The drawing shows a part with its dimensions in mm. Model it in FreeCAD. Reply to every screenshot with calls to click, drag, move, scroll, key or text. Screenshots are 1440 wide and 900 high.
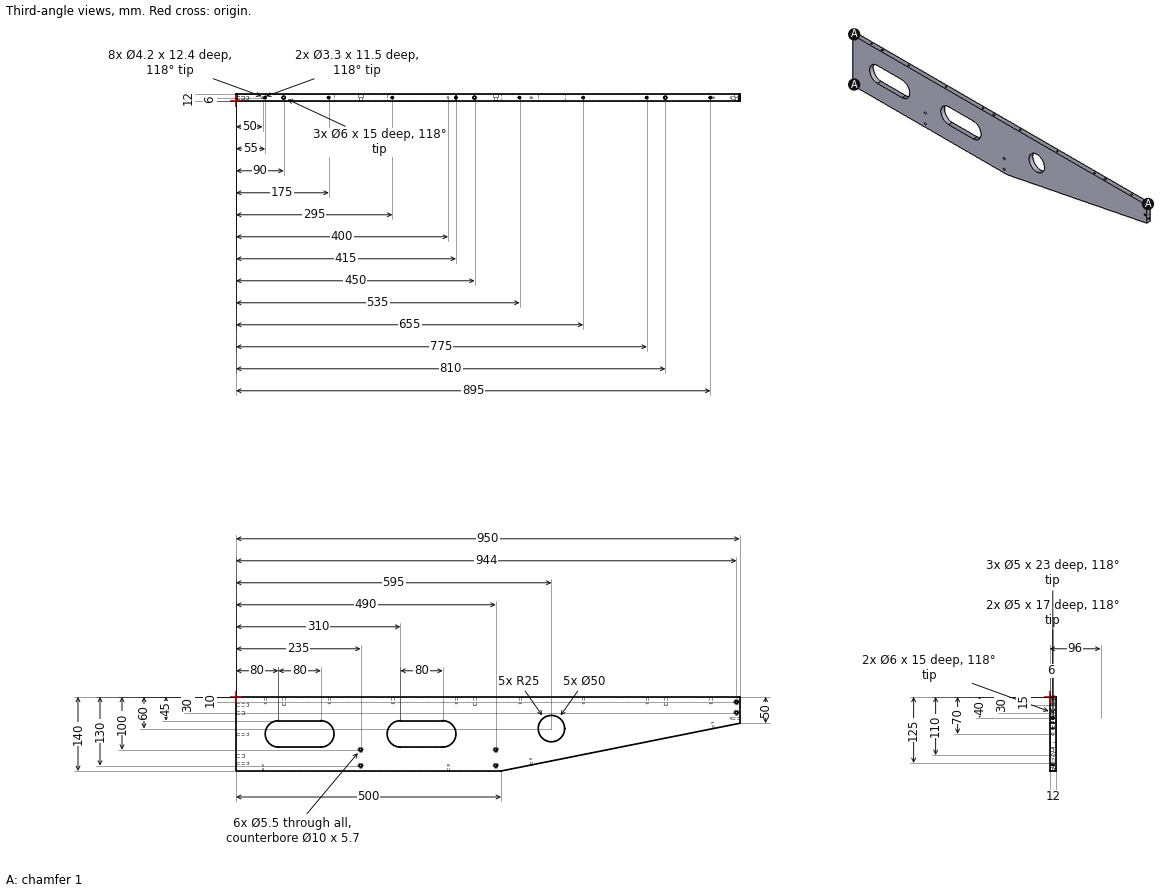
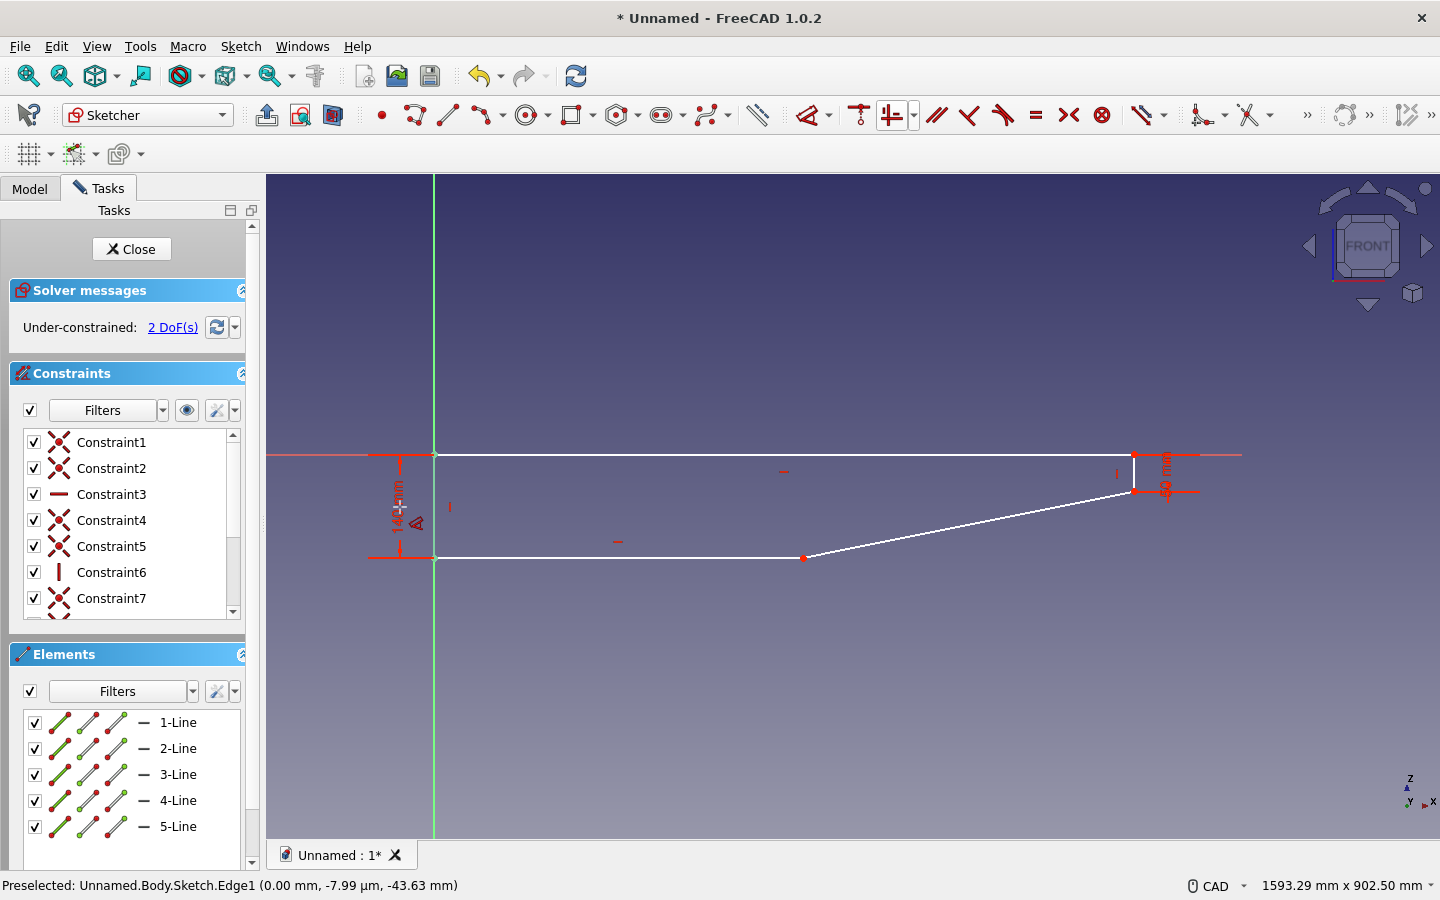
click(545, 558)
click(619, 592)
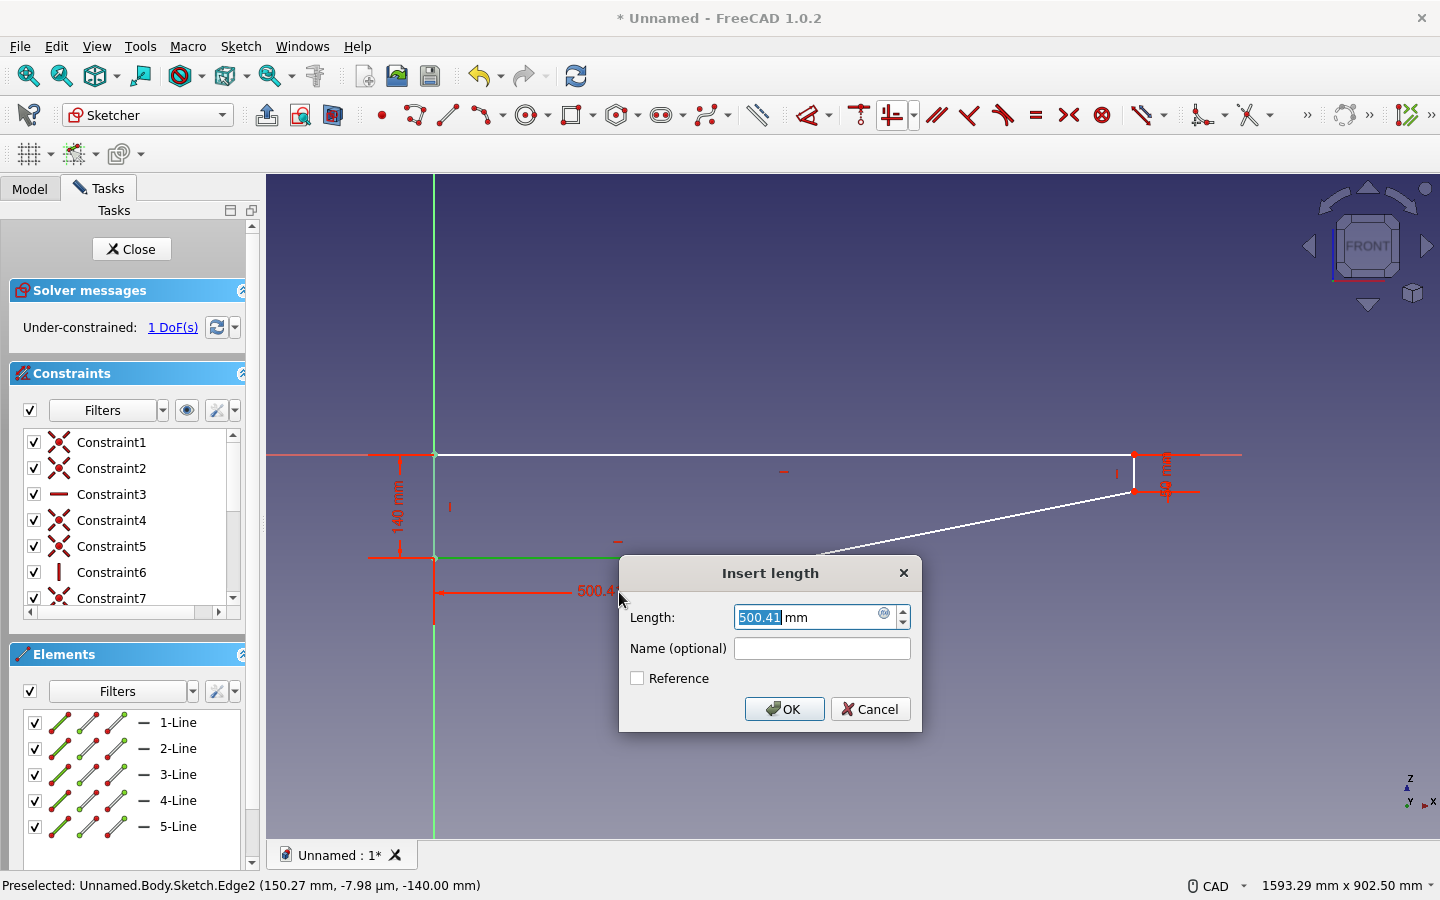
text(500)
key(Return)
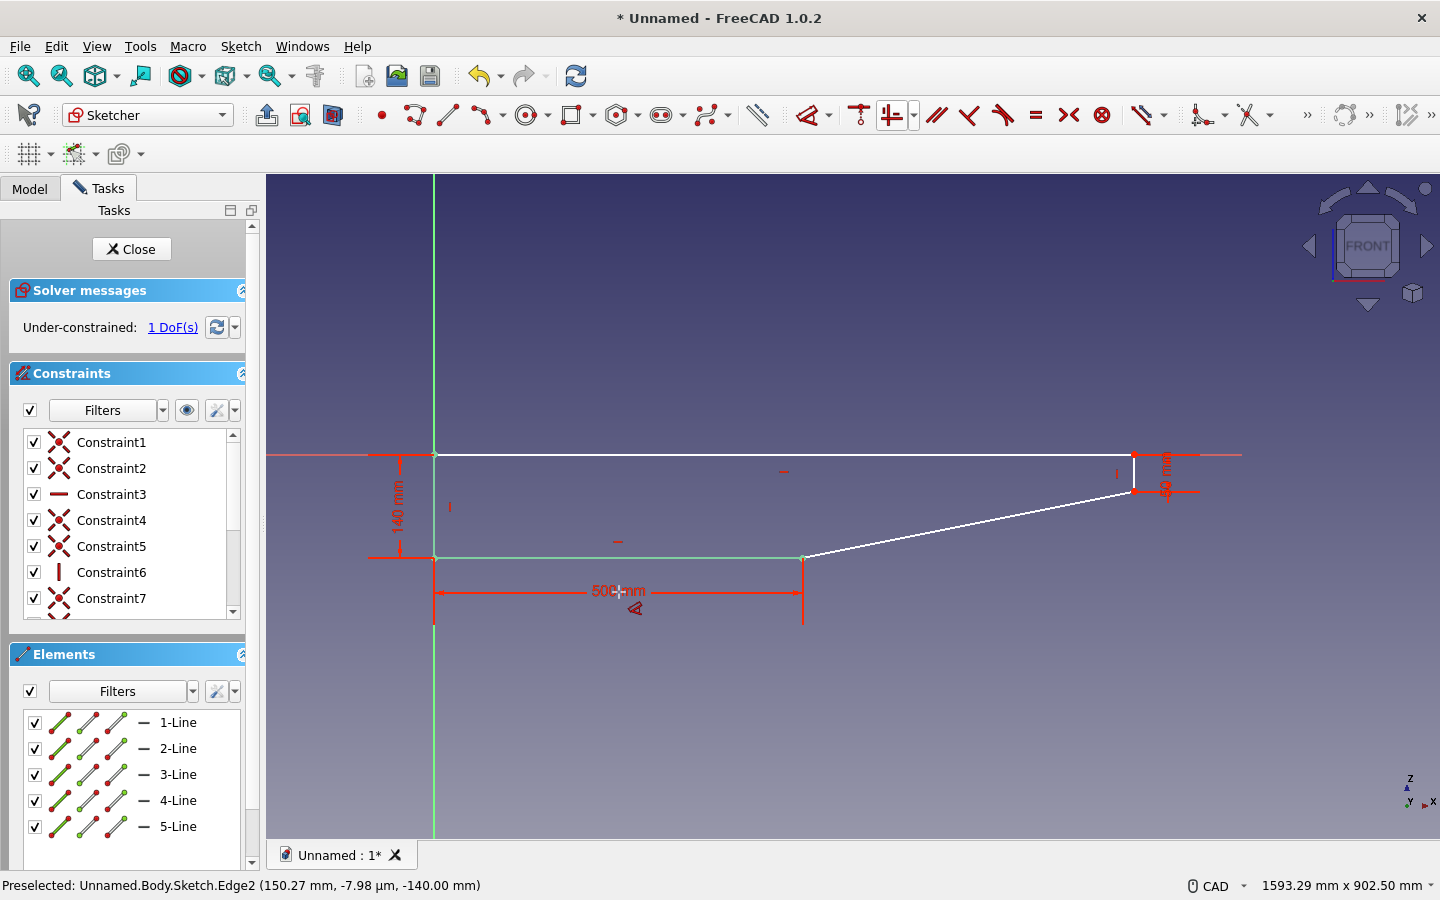
click(924, 455)
click(784, 421)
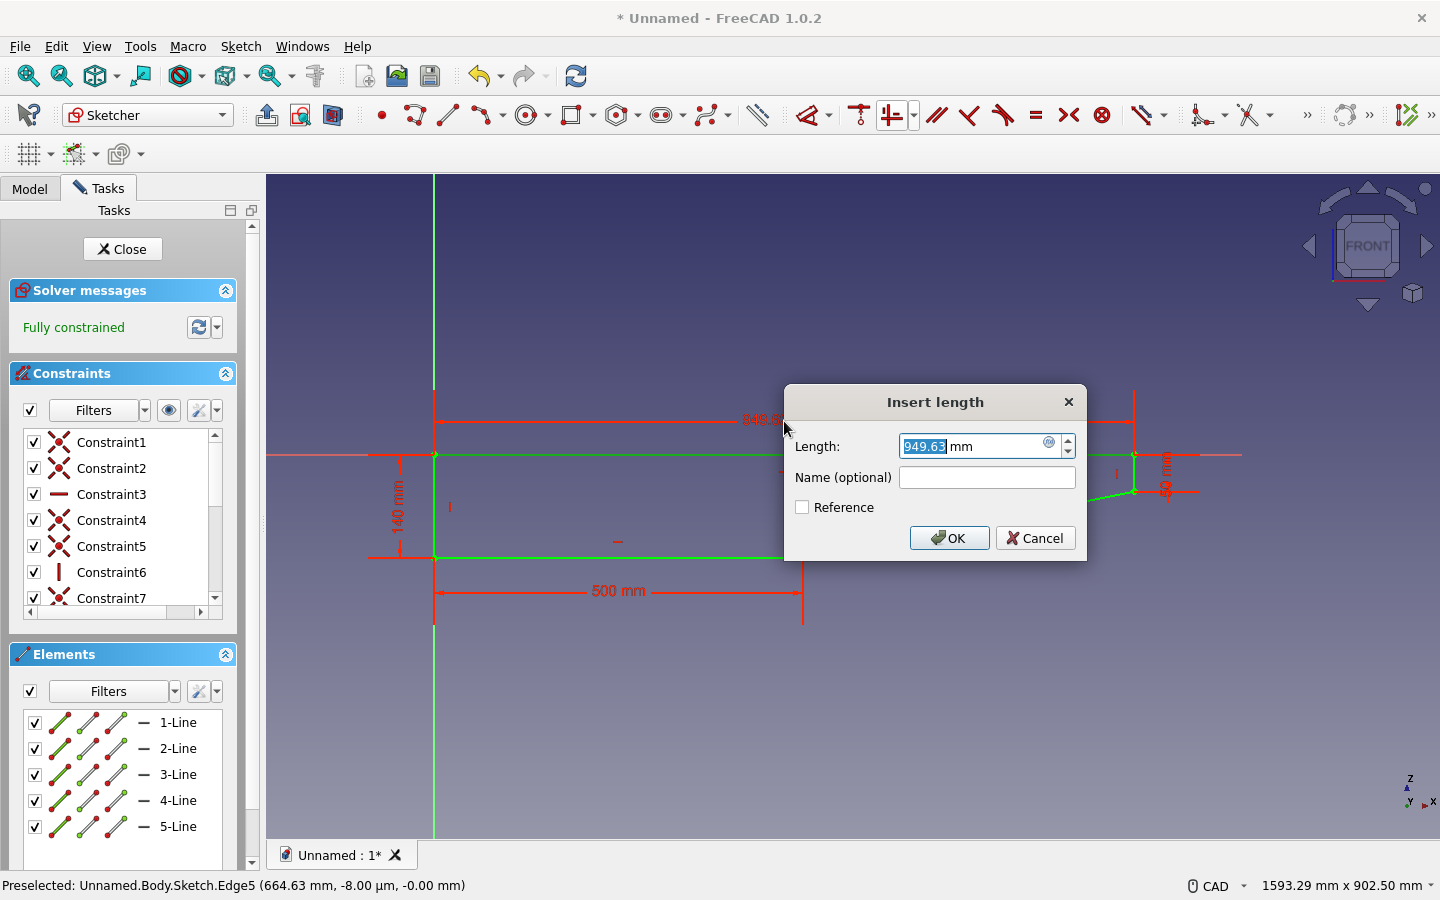
text(950)
key(Return)
key(Escape)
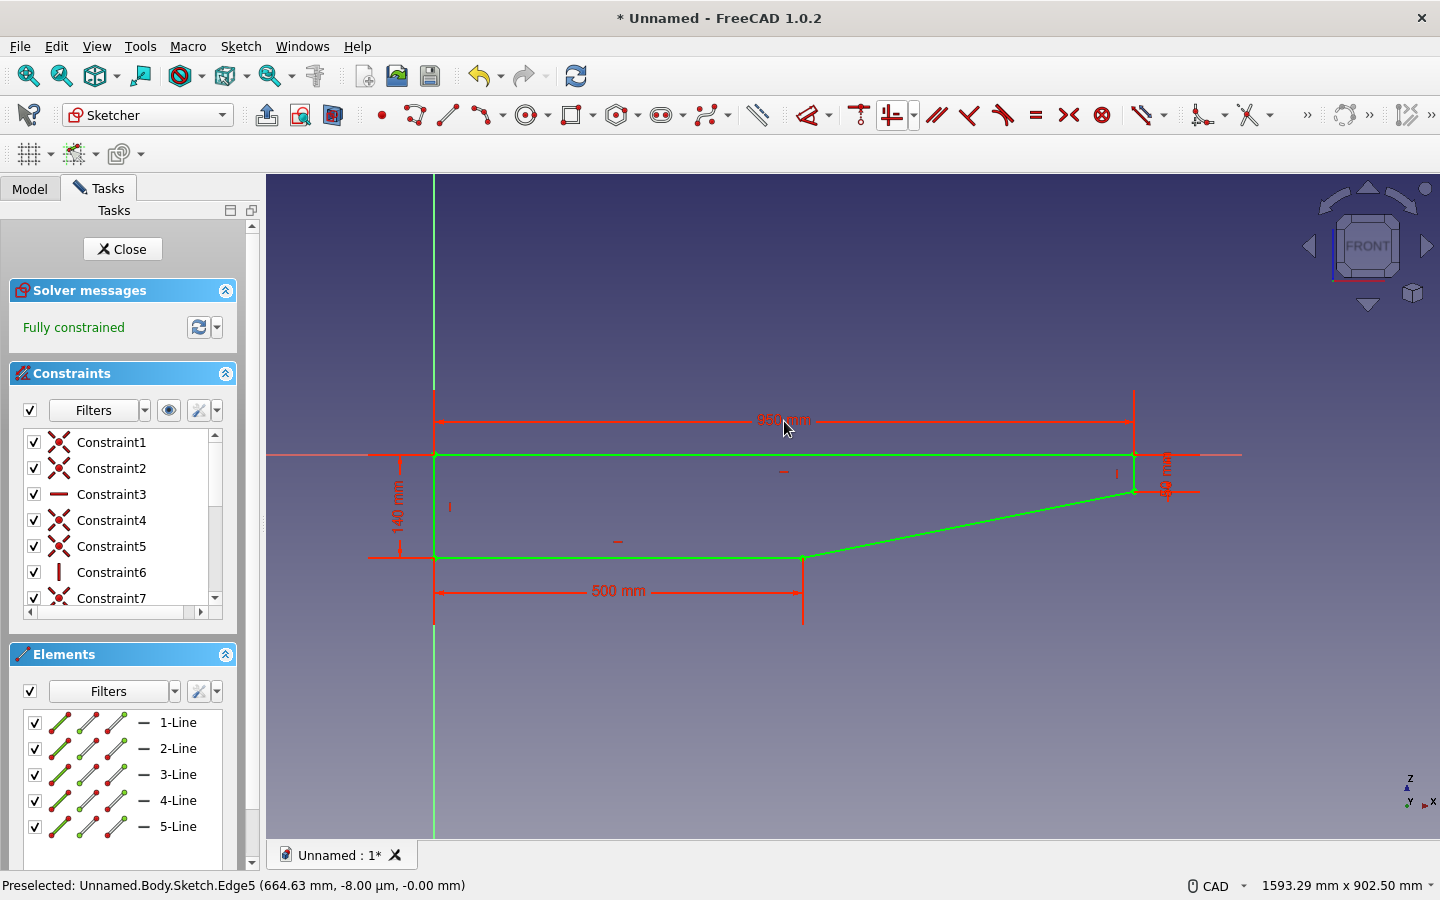
click(123, 249)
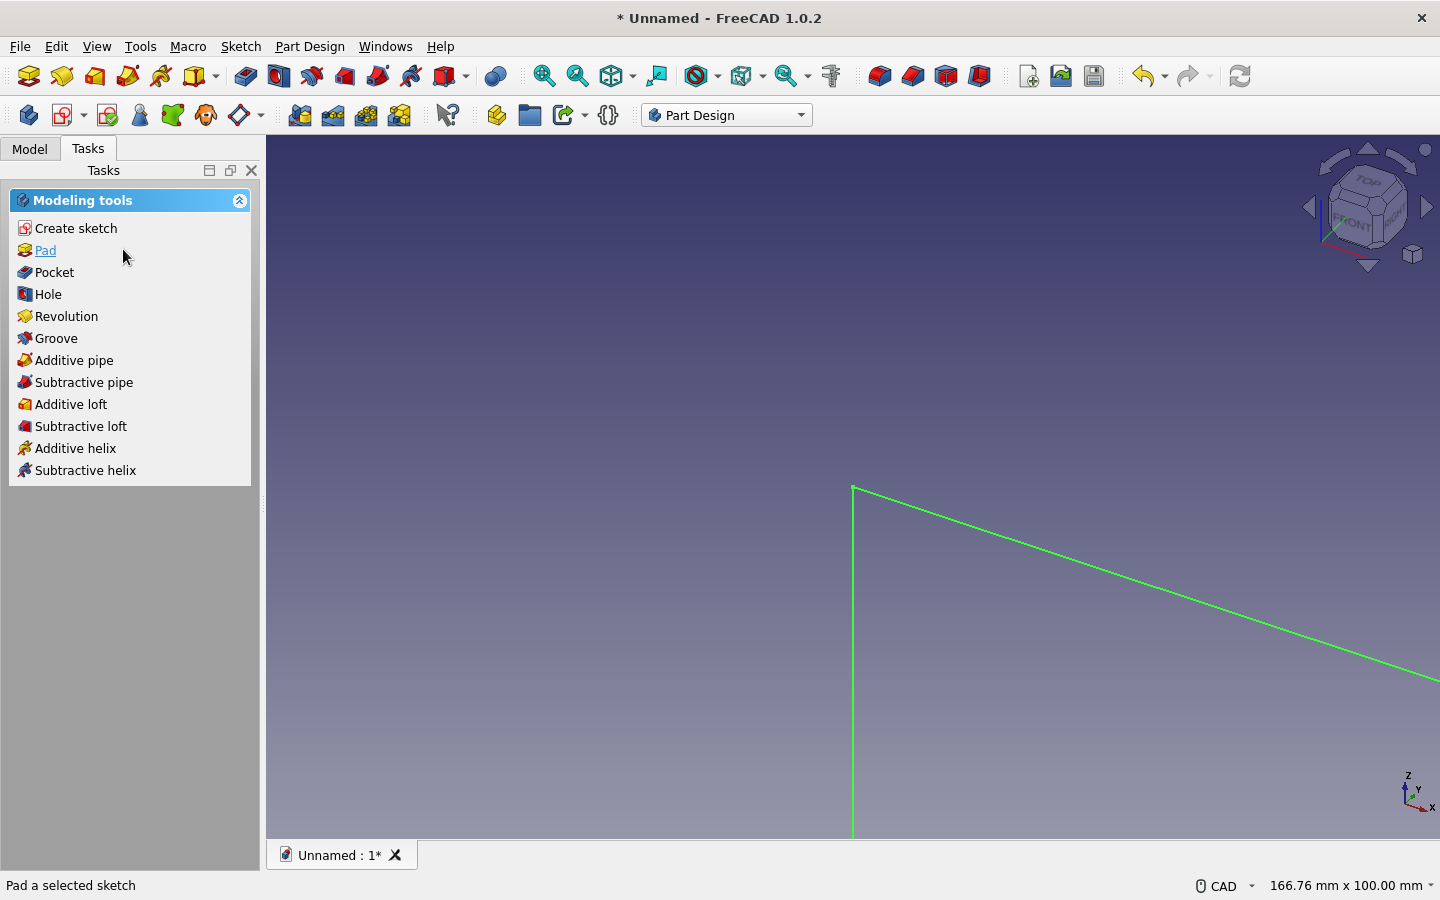
click(29, 76)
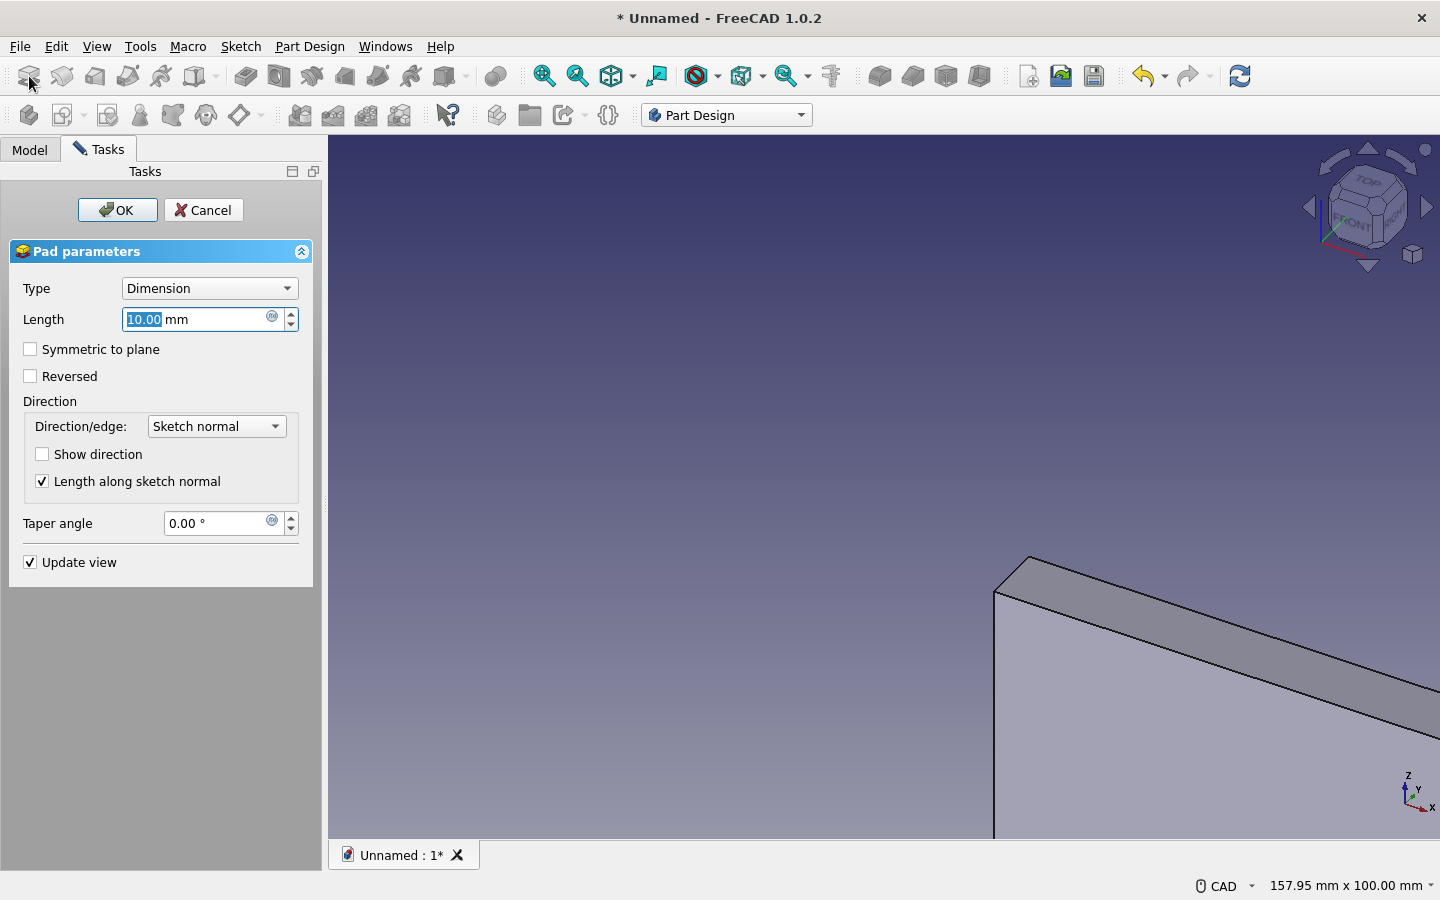
text(12)
key(Tab)